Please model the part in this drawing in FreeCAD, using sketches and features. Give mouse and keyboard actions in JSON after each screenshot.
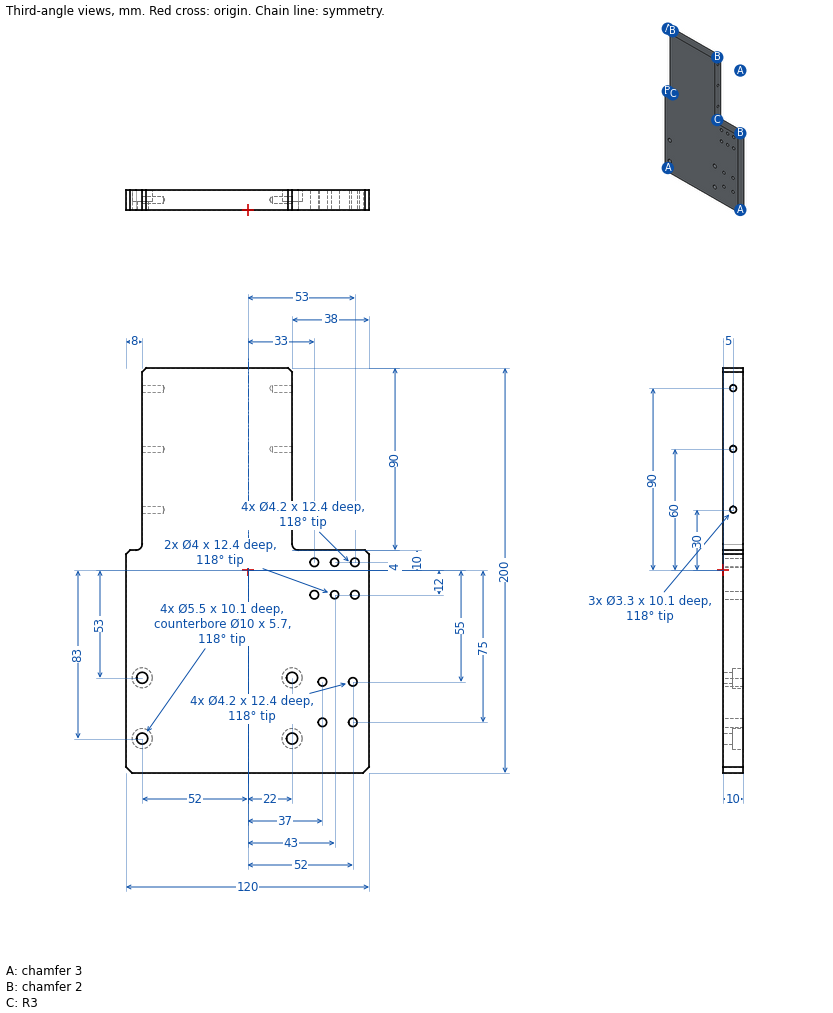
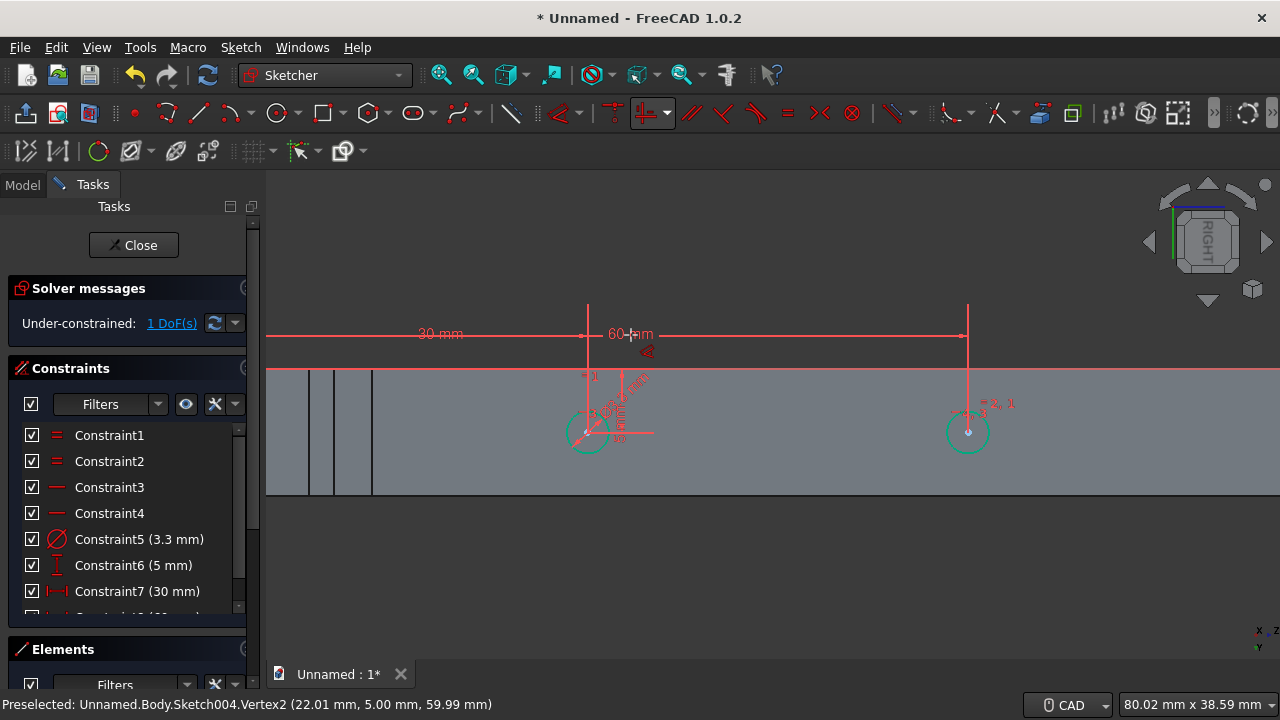
{"action": "scroll", "coordinate": [602, 418], "scroll_direction": "down", "scroll_amount": 3}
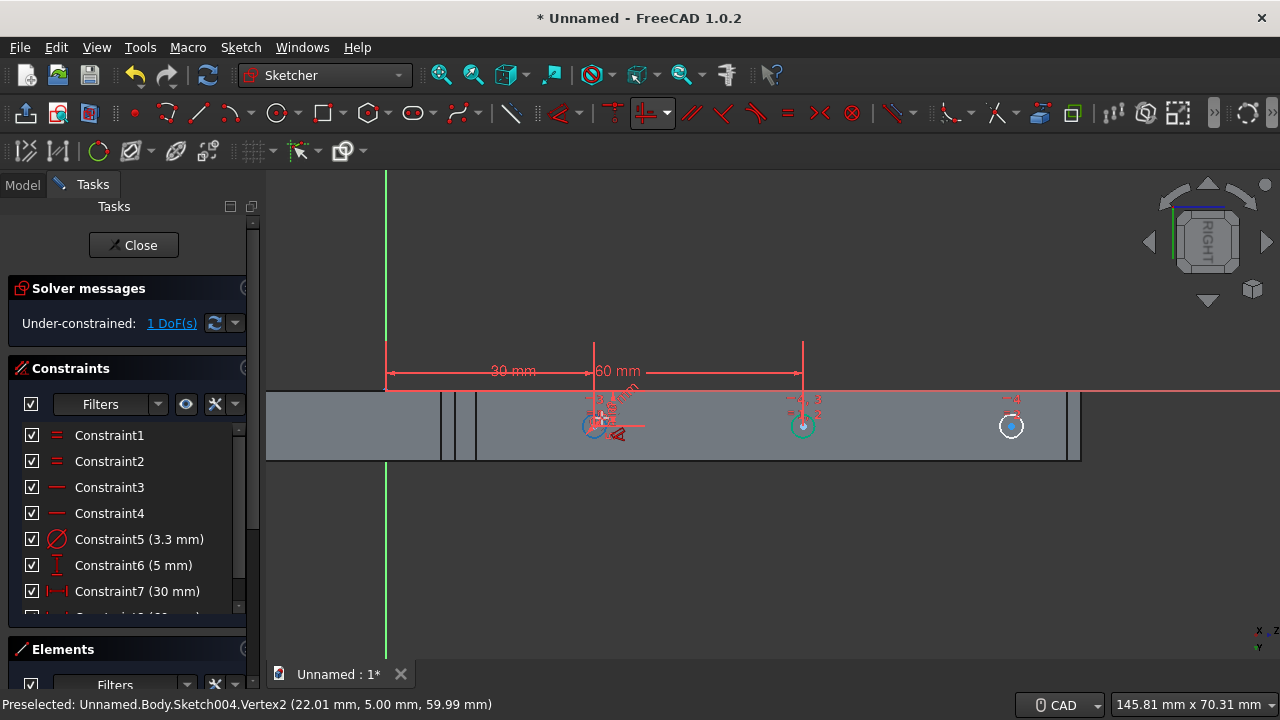
{"action": "left_click", "coordinate": [1012, 426]}
{"action": "left_click", "coordinate": [699, 357]}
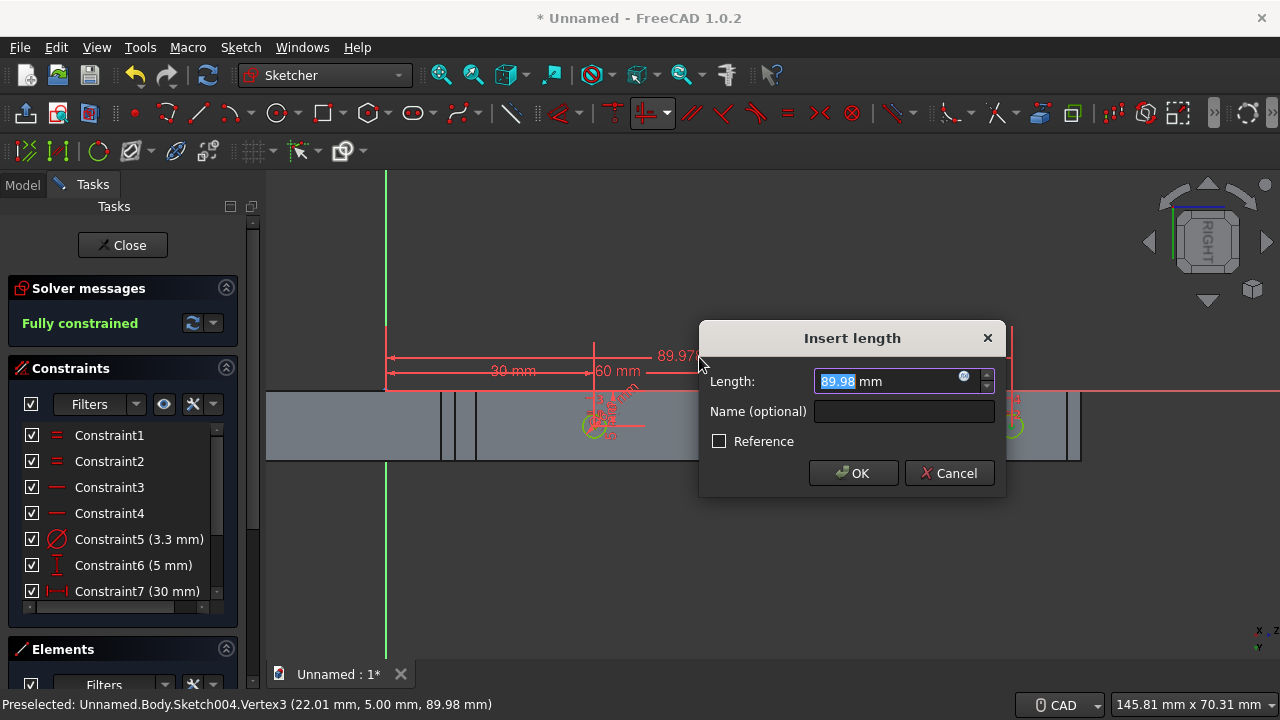
{"action": "type", "text": "90"}
{"action": "key", "text": "Return"}
{"action": "key", "text": "Escape"}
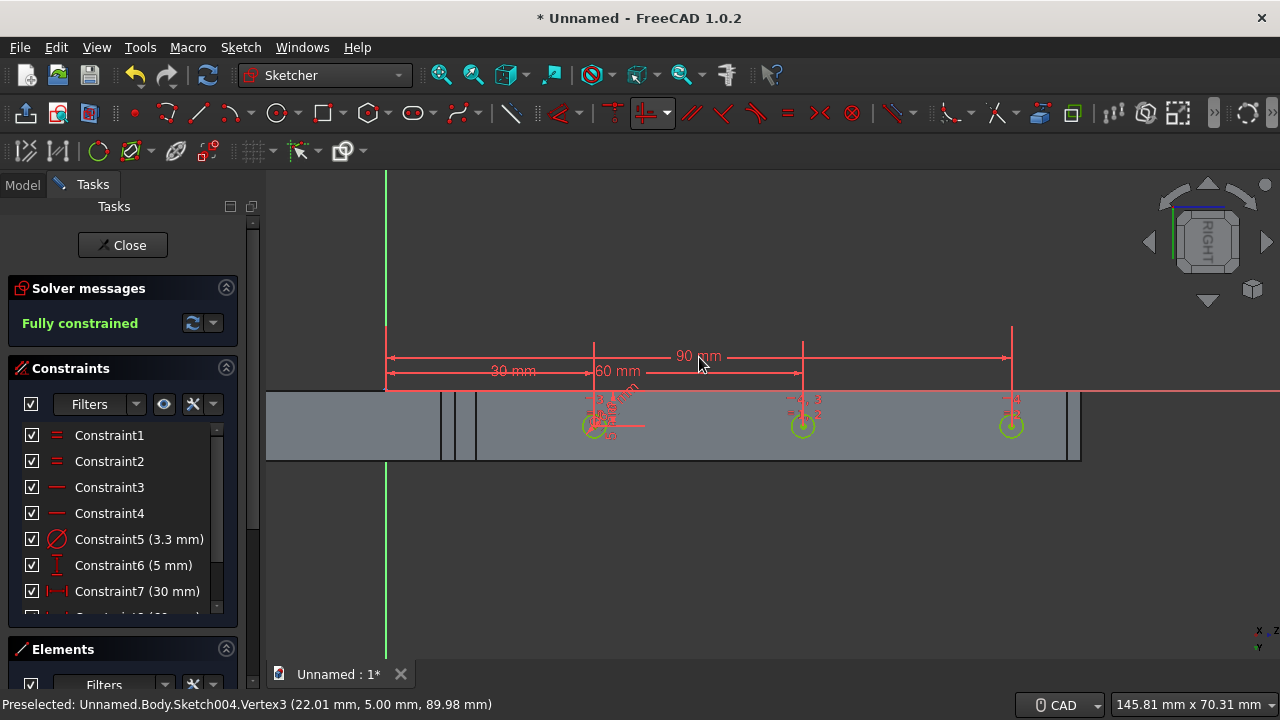
{"action": "left_click", "coordinate": [123, 245]}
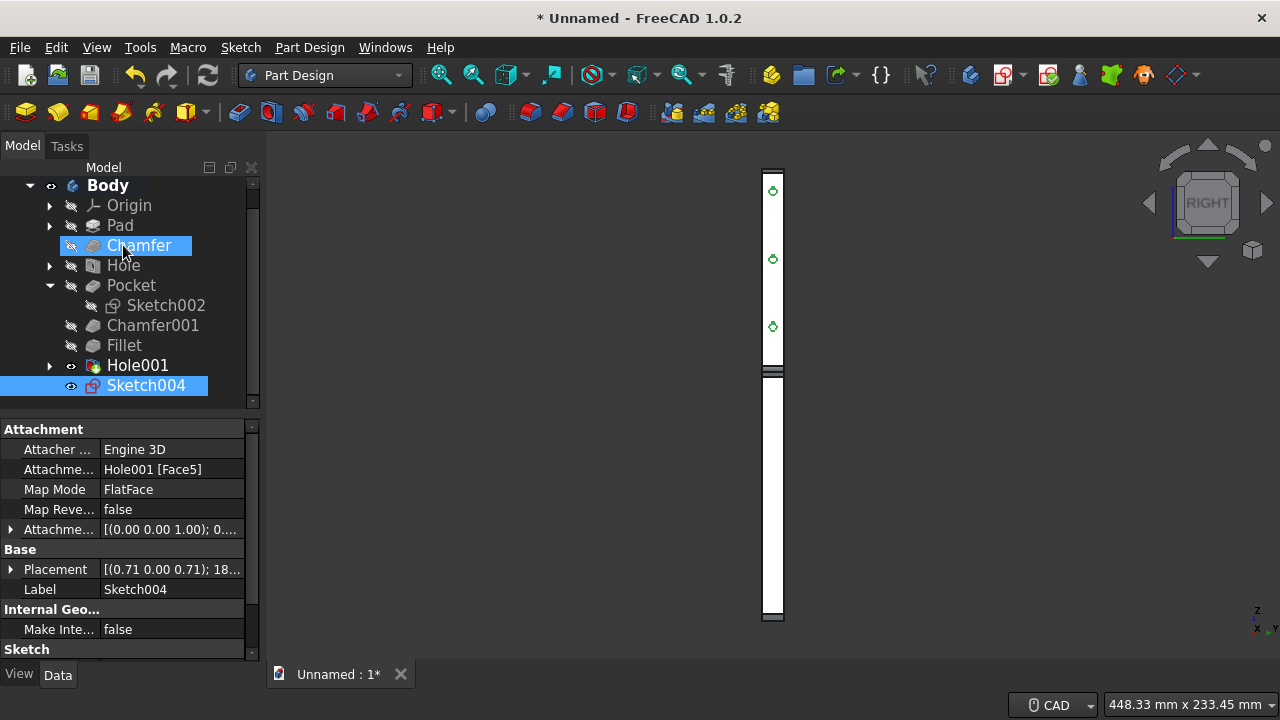
{"action": "left_click", "coordinate": [272, 112]}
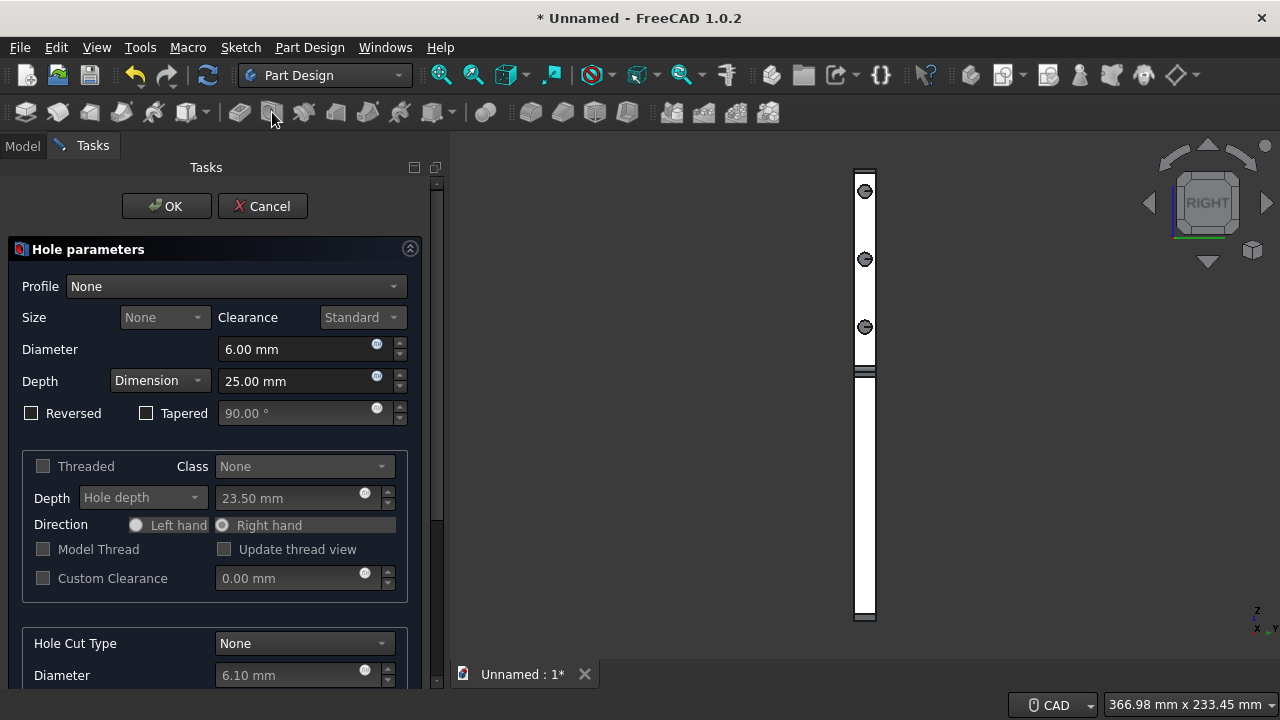
{"action": "triple_click", "coordinate": [305, 349]}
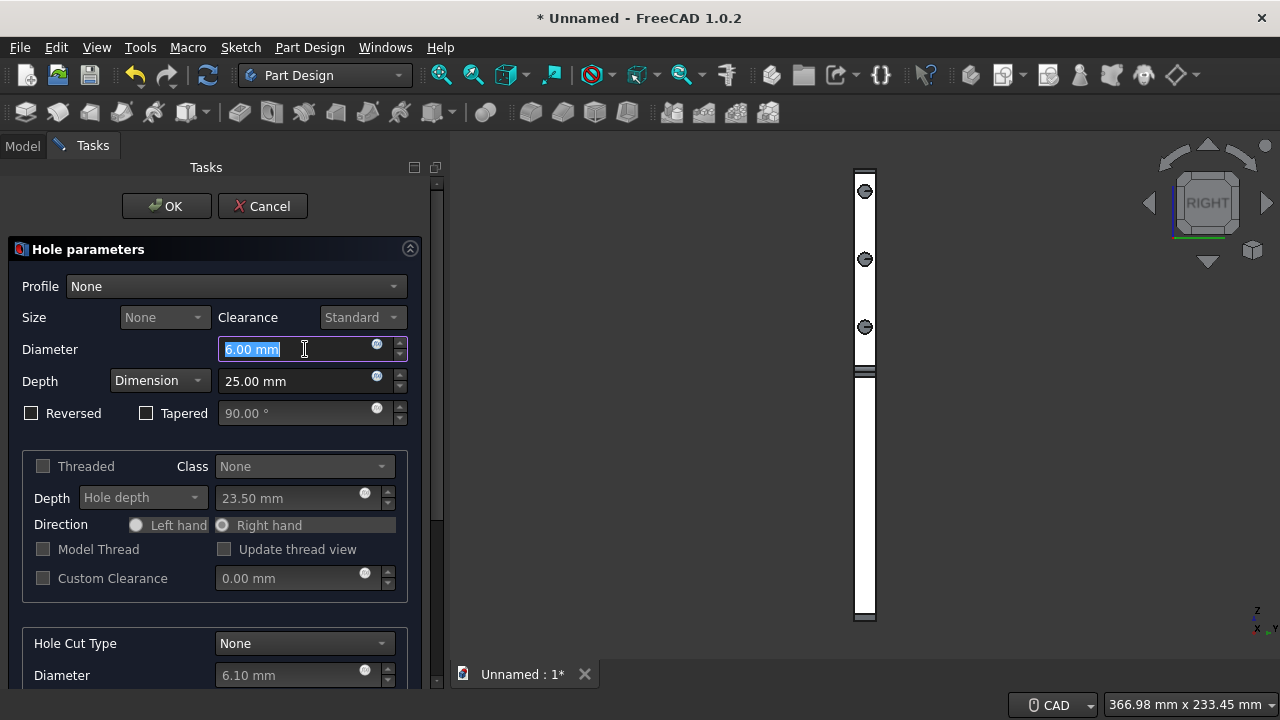
{"action": "type", "text": "3.3"}
{"action": "key", "text": "Tab"}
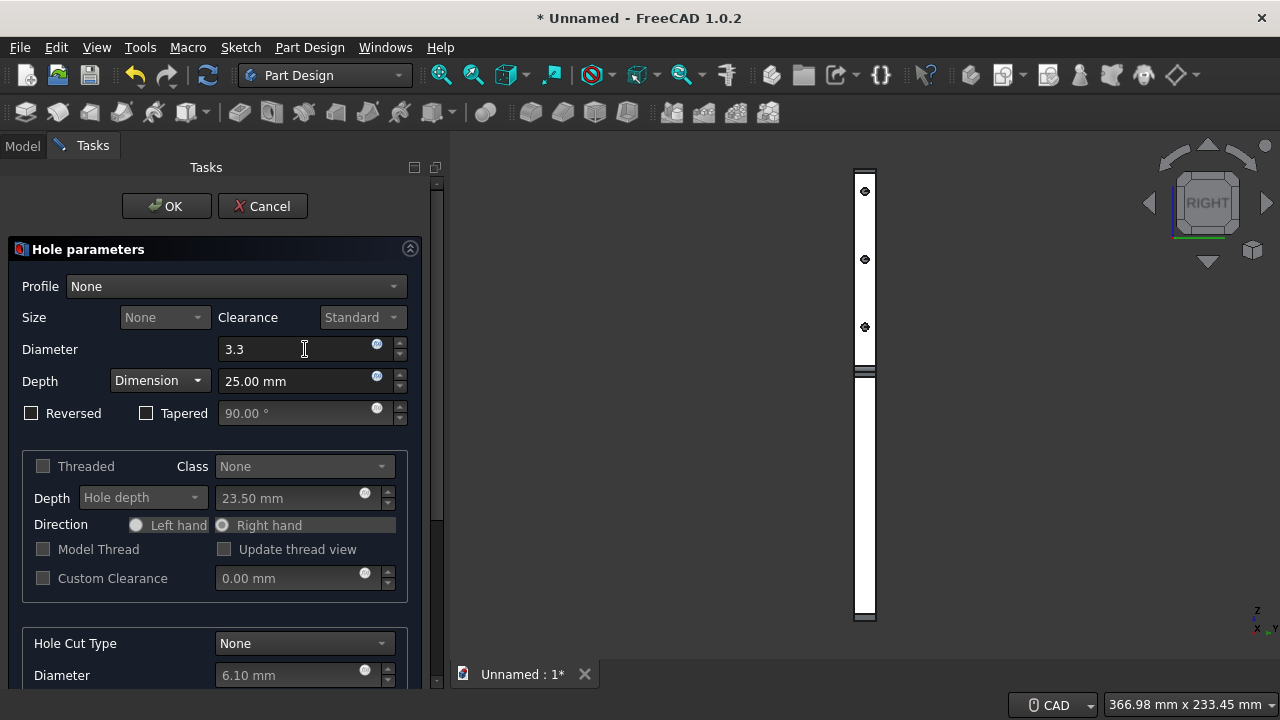
{"action": "triple_click", "coordinate": [305, 381]}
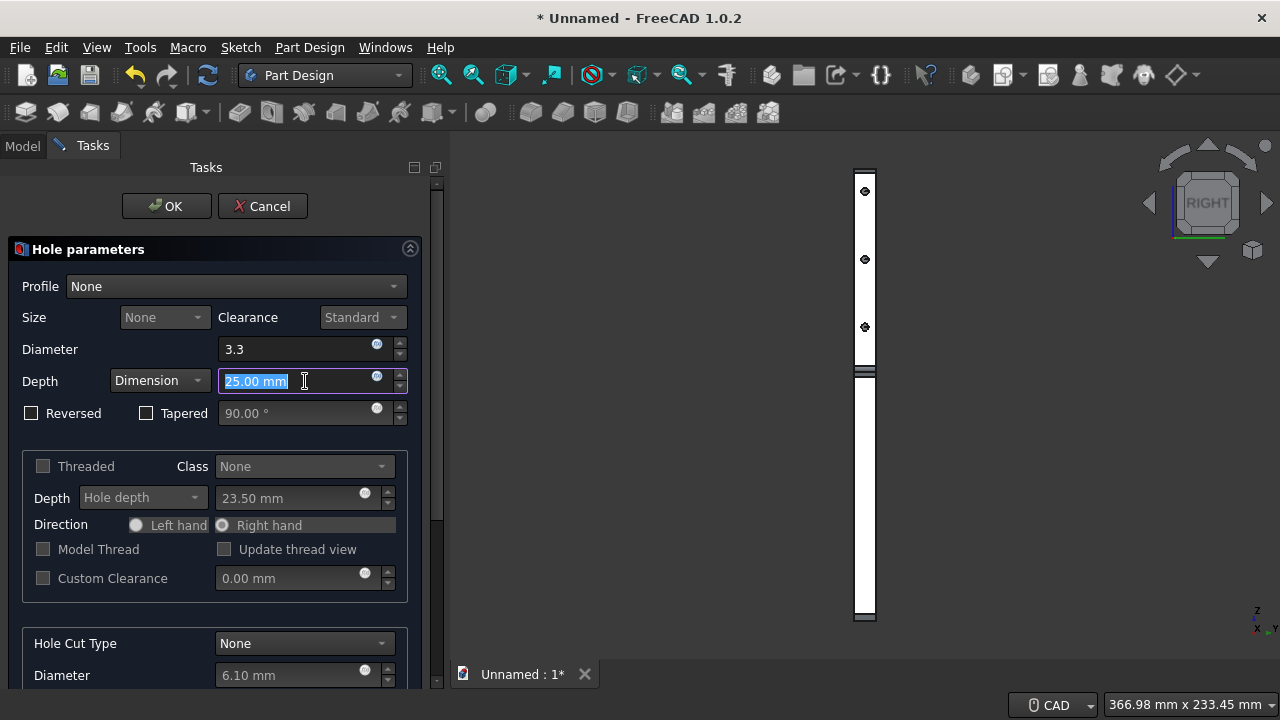
{"action": "type", "text": "10.1"}
{"action": "key", "text": "Tab"}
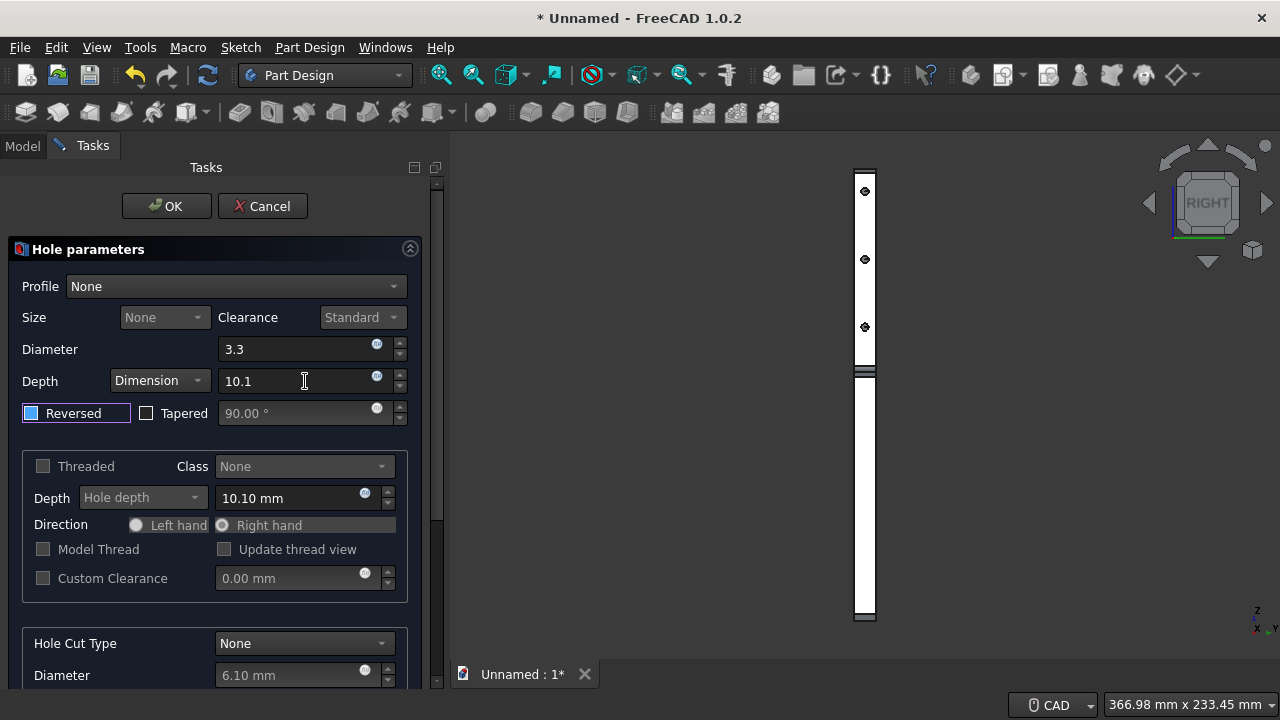
{"action": "left_click", "coordinate": [167, 206]}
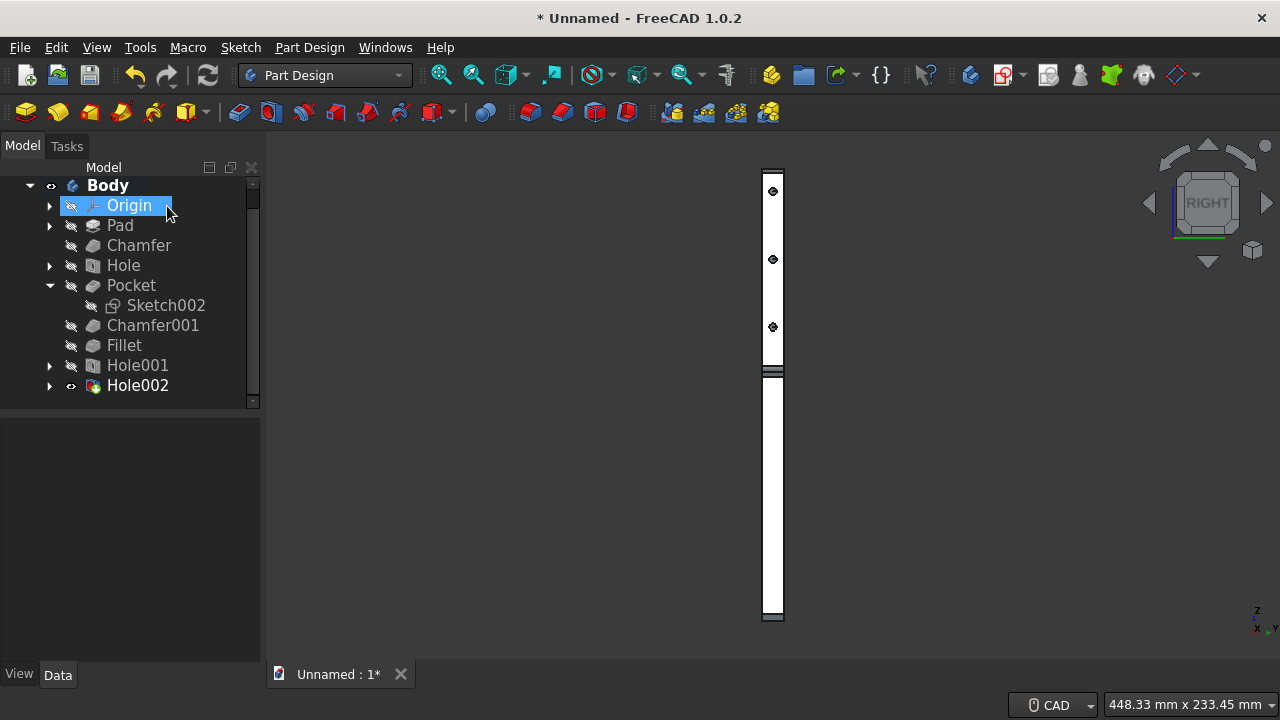
{"action": "key", "text": "4"}